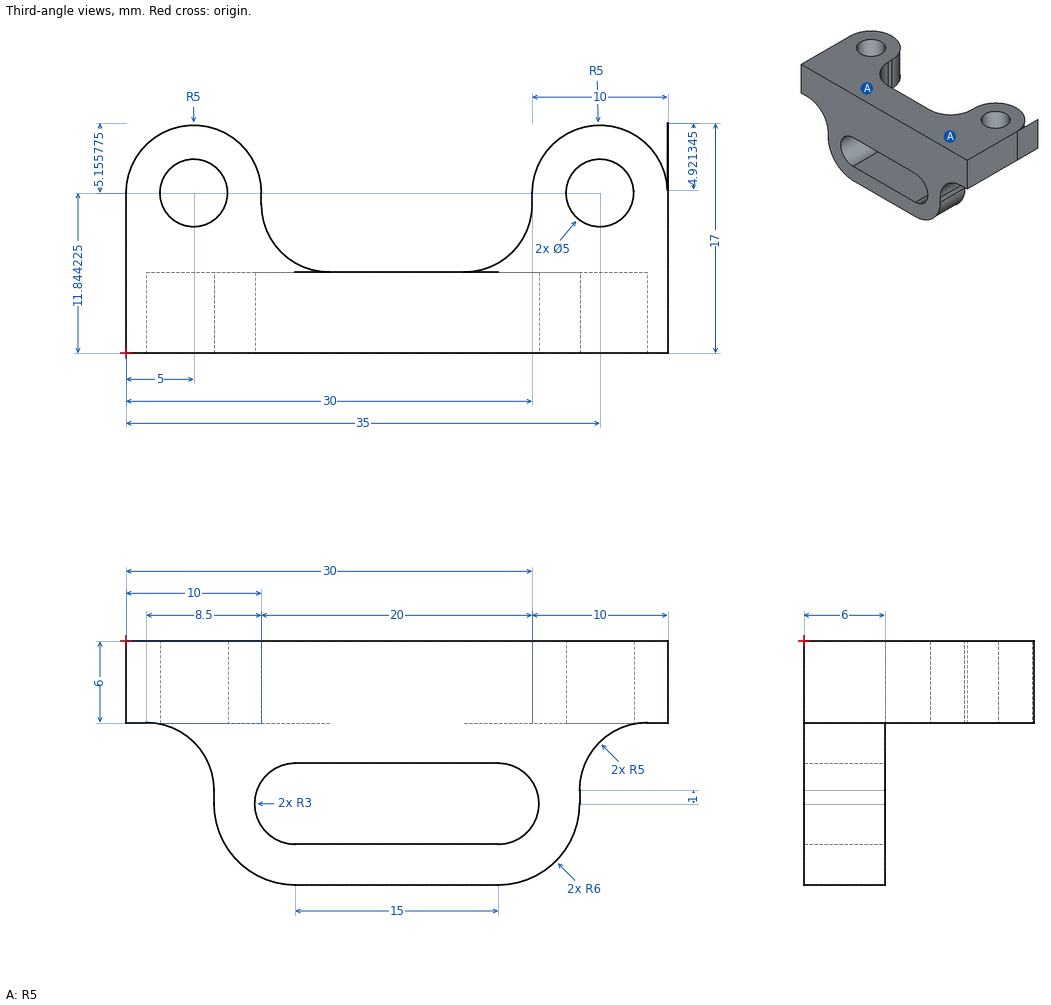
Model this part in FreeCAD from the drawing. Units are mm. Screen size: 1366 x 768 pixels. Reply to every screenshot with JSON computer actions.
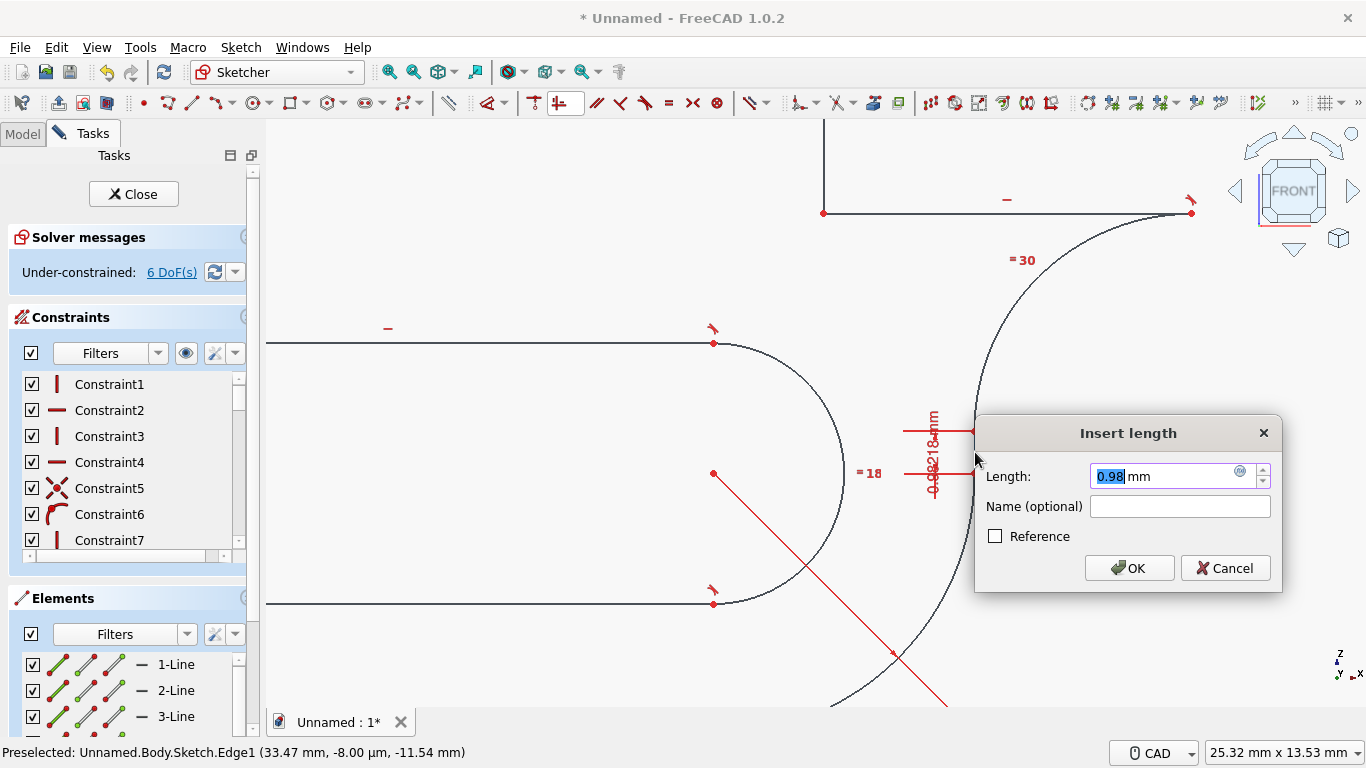
{"action": "type", "text": "1"}
{"action": "key", "text": "Return"}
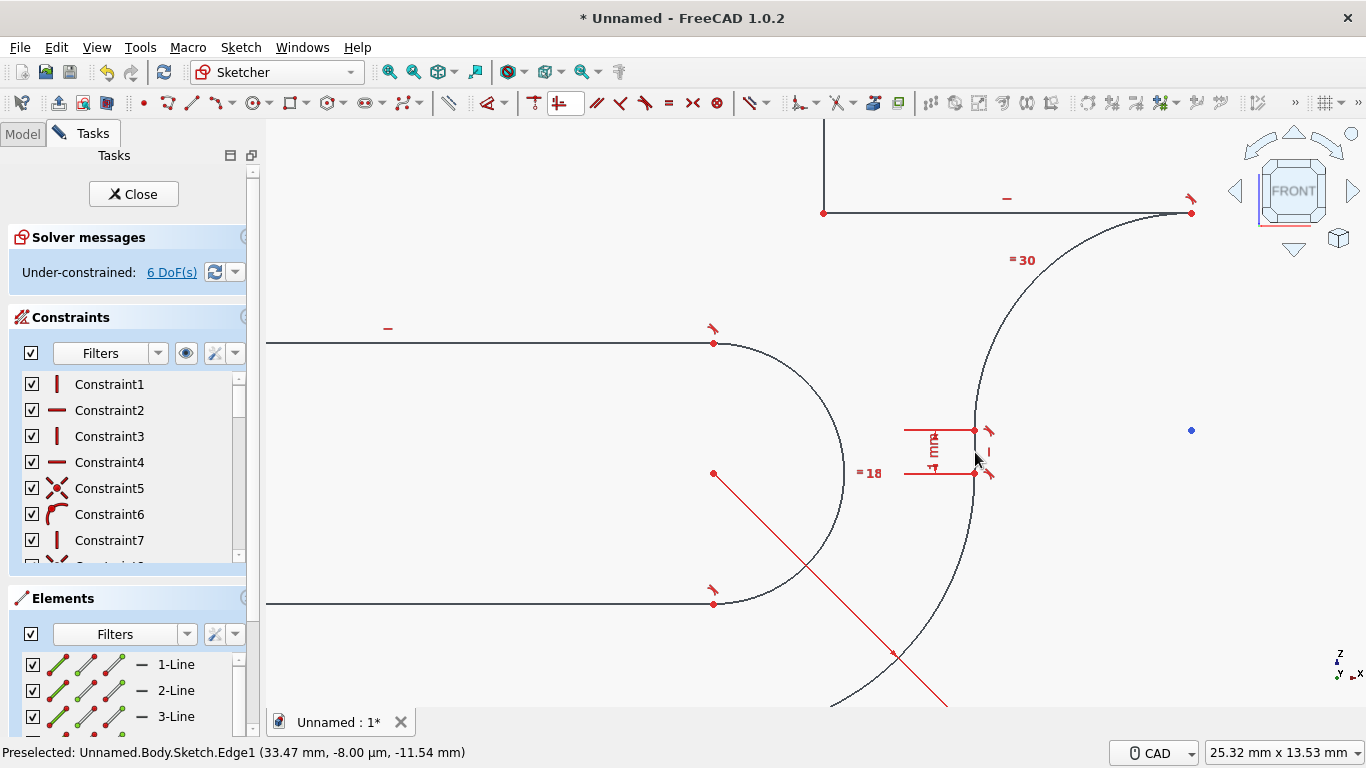
{"action": "scroll", "coordinate": [975, 454], "scroll_direction": "down", "scroll_amount": 5}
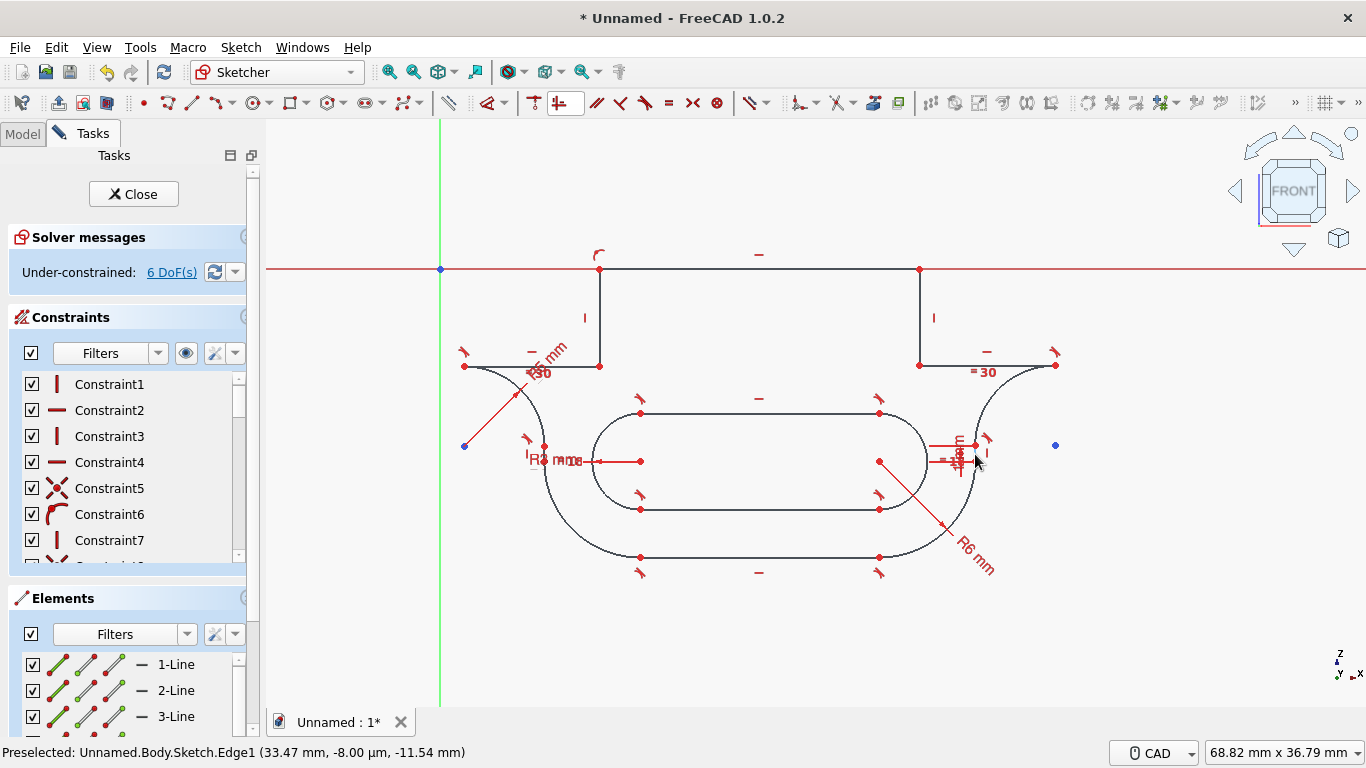
{"action": "scroll", "coordinate": [544, 457], "scroll_direction": "up", "scroll_amount": 6}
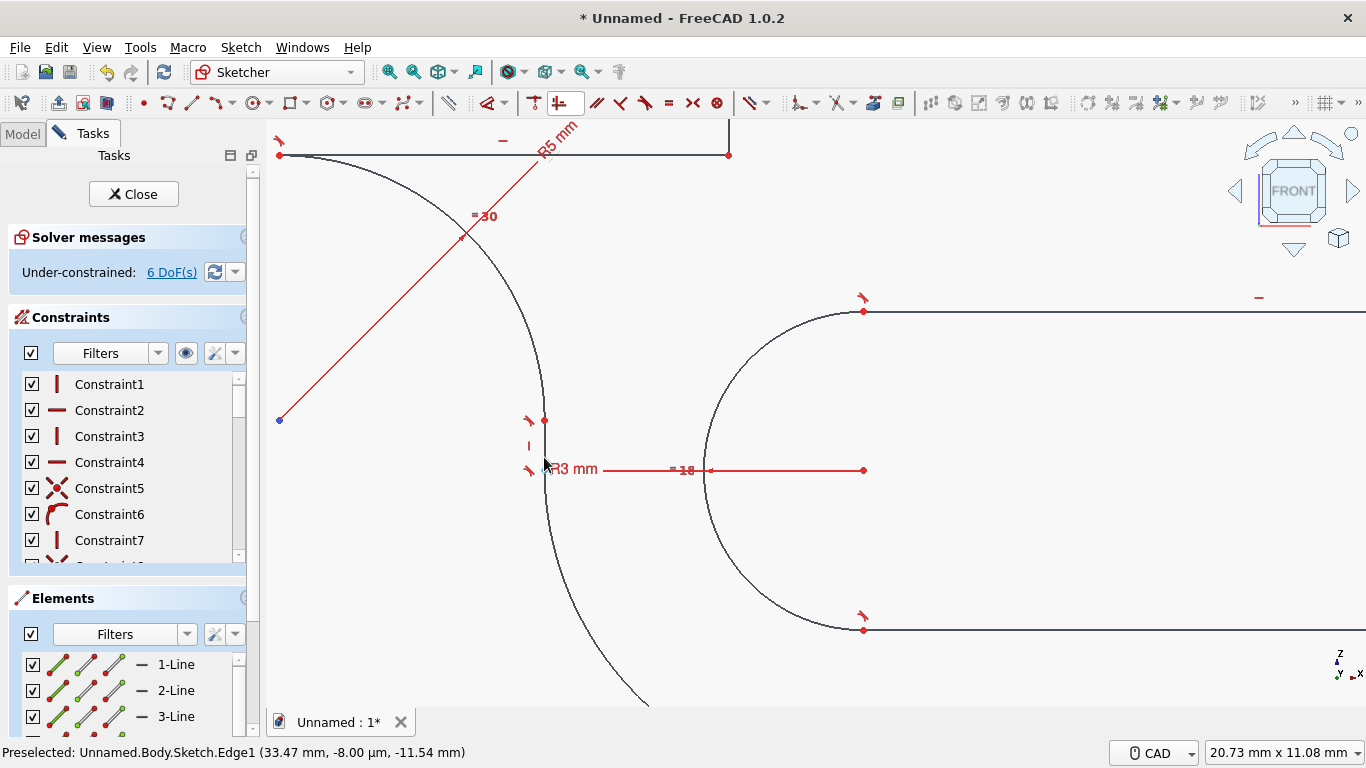
{"action": "left_click", "coordinate": [545, 456]}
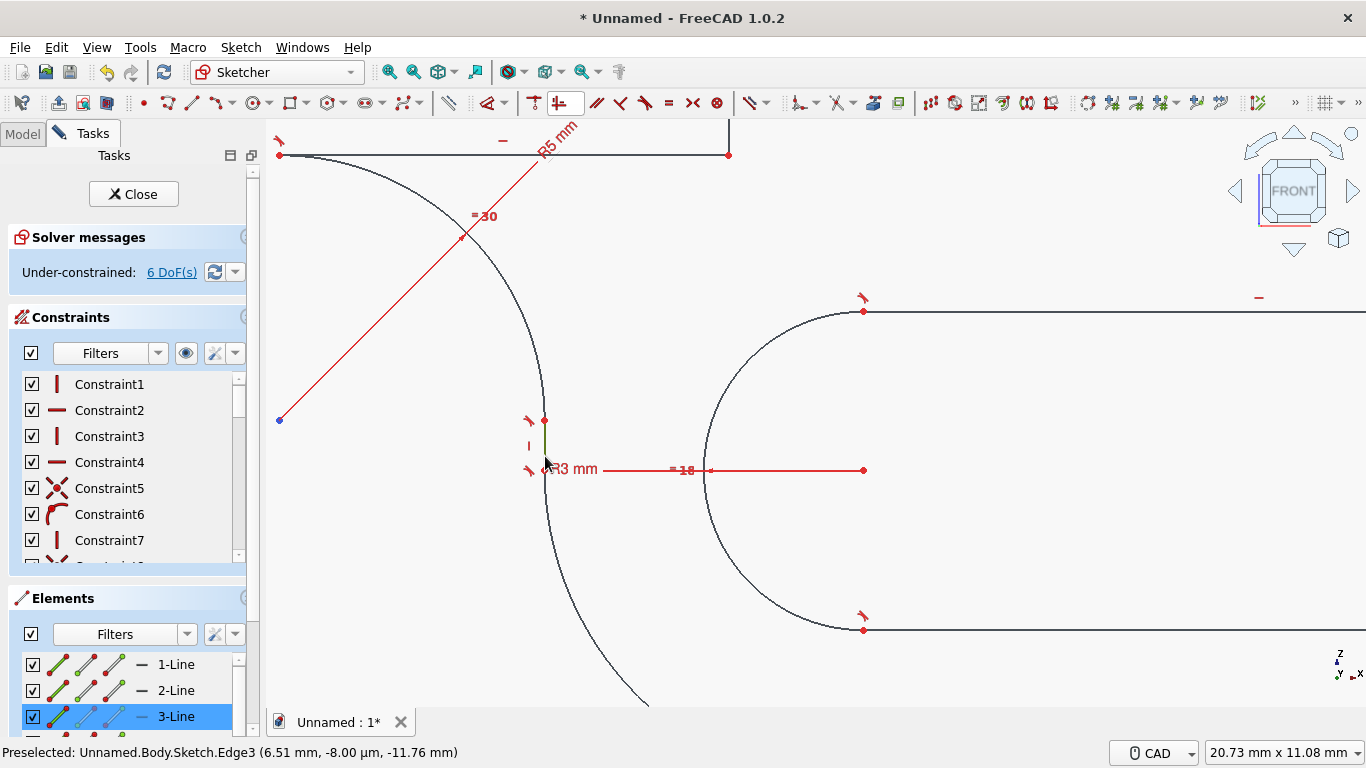
{"action": "key", "text": "i"}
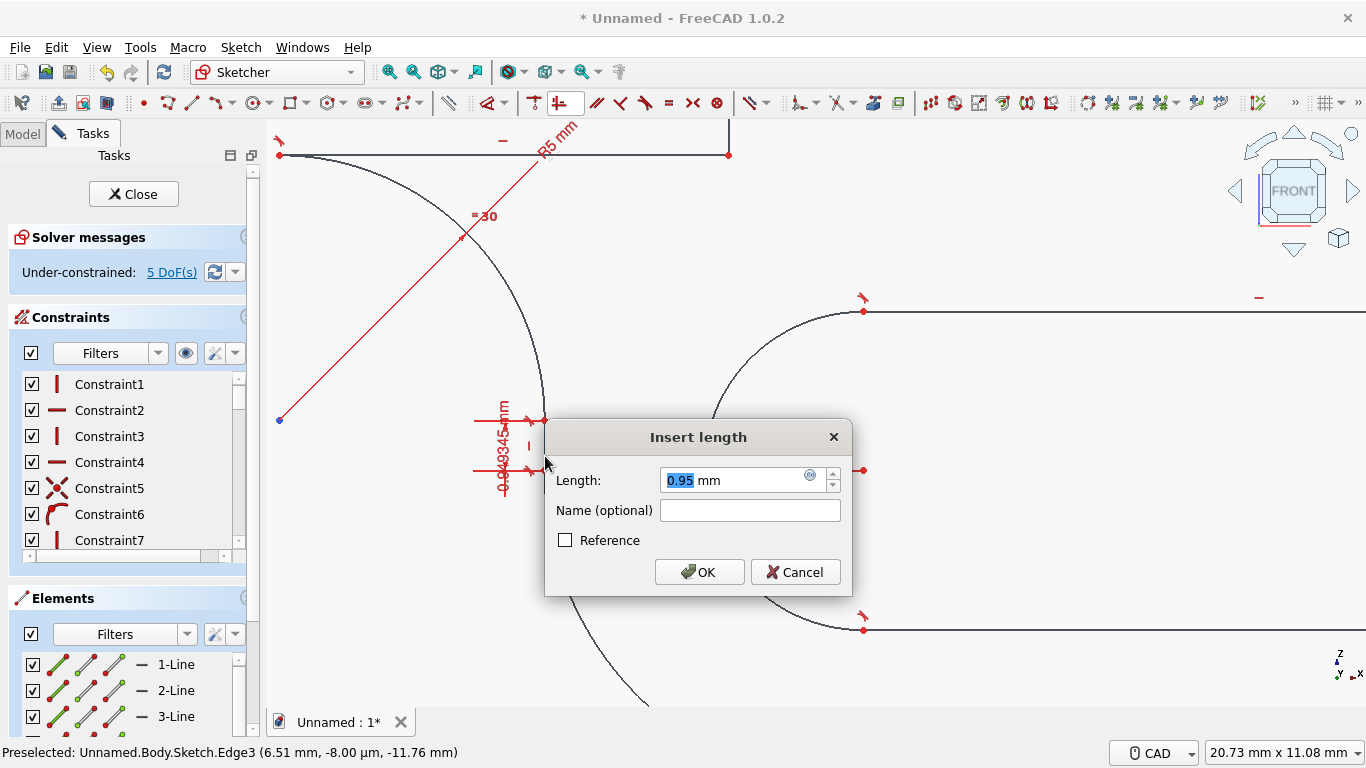
{"action": "type", "text": "1"}
{"action": "key", "text": "Return"}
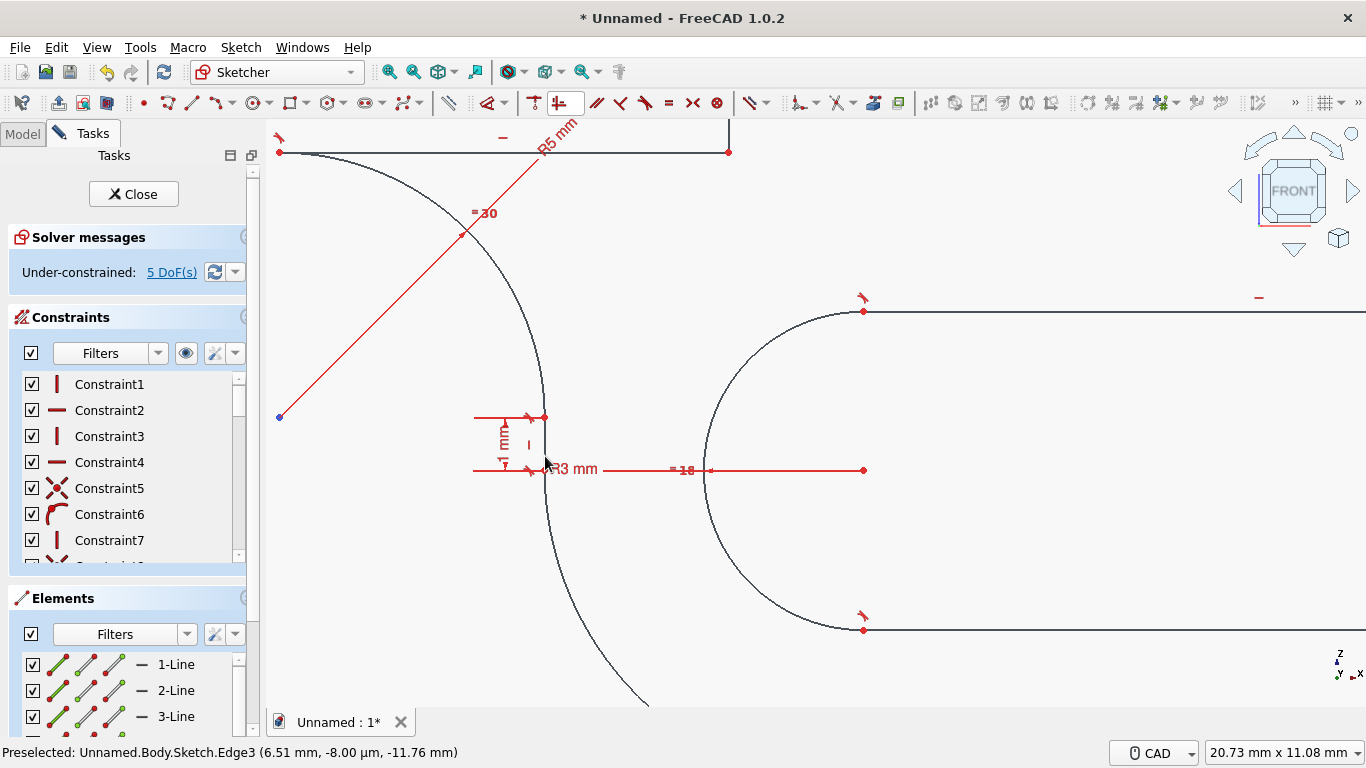
{"action": "scroll", "coordinate": [544, 457], "scroll_direction": "down", "scroll_amount": 6}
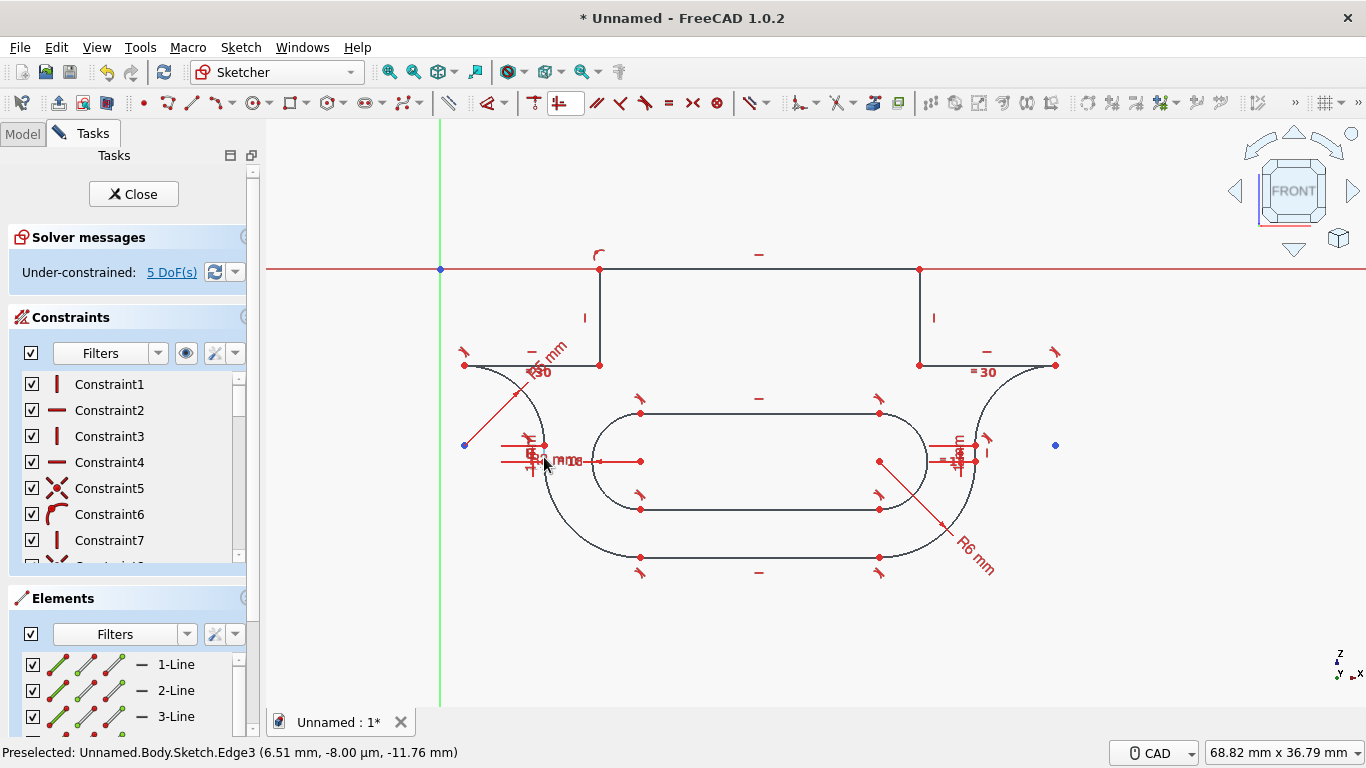
{"action": "left_click", "coordinate": [600, 337]}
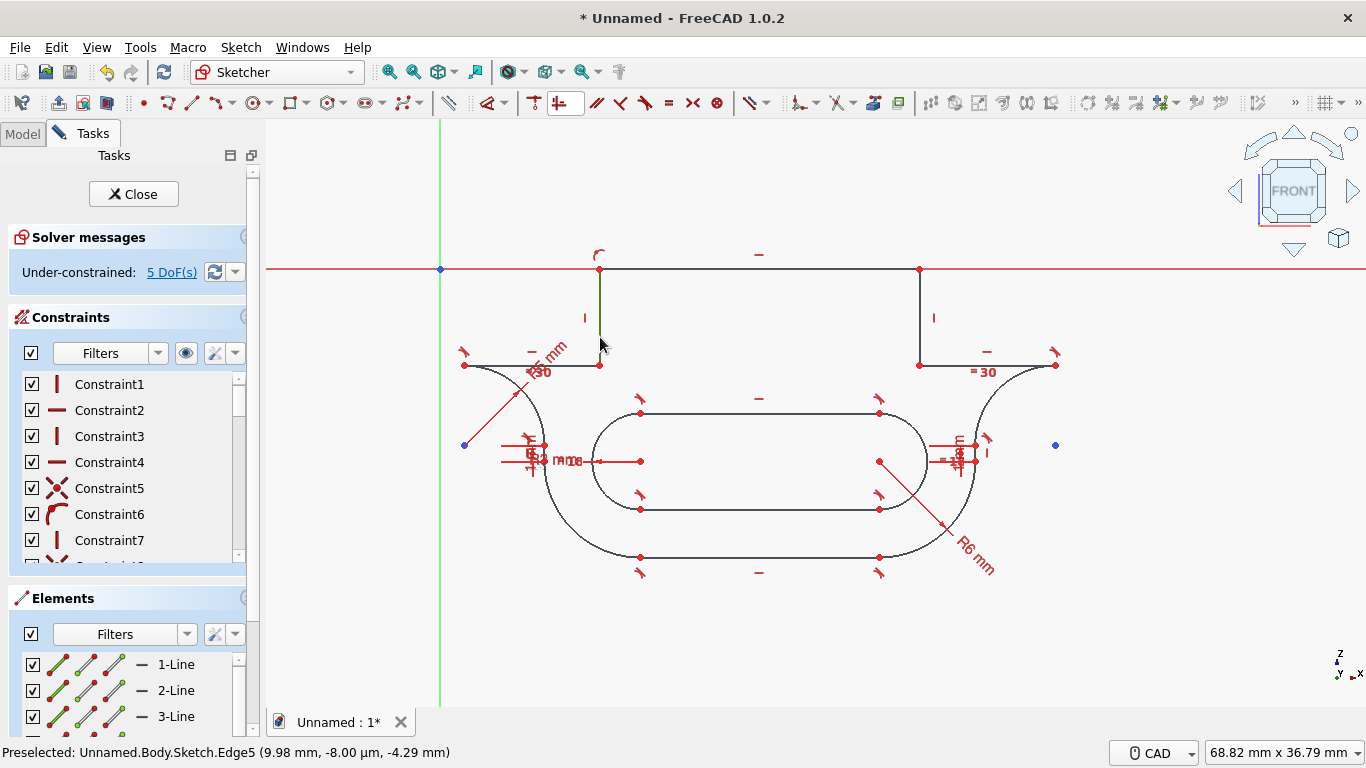
{"action": "key", "text": "i"}